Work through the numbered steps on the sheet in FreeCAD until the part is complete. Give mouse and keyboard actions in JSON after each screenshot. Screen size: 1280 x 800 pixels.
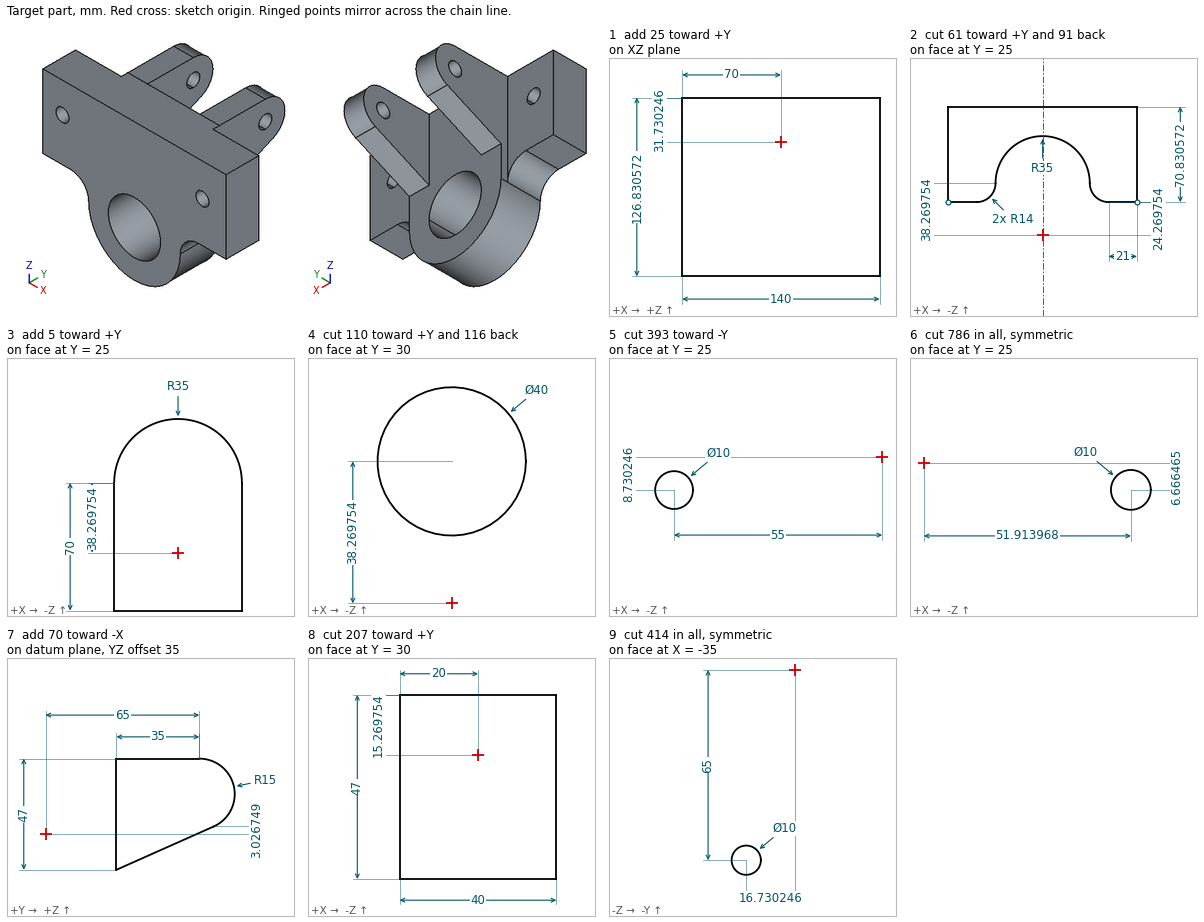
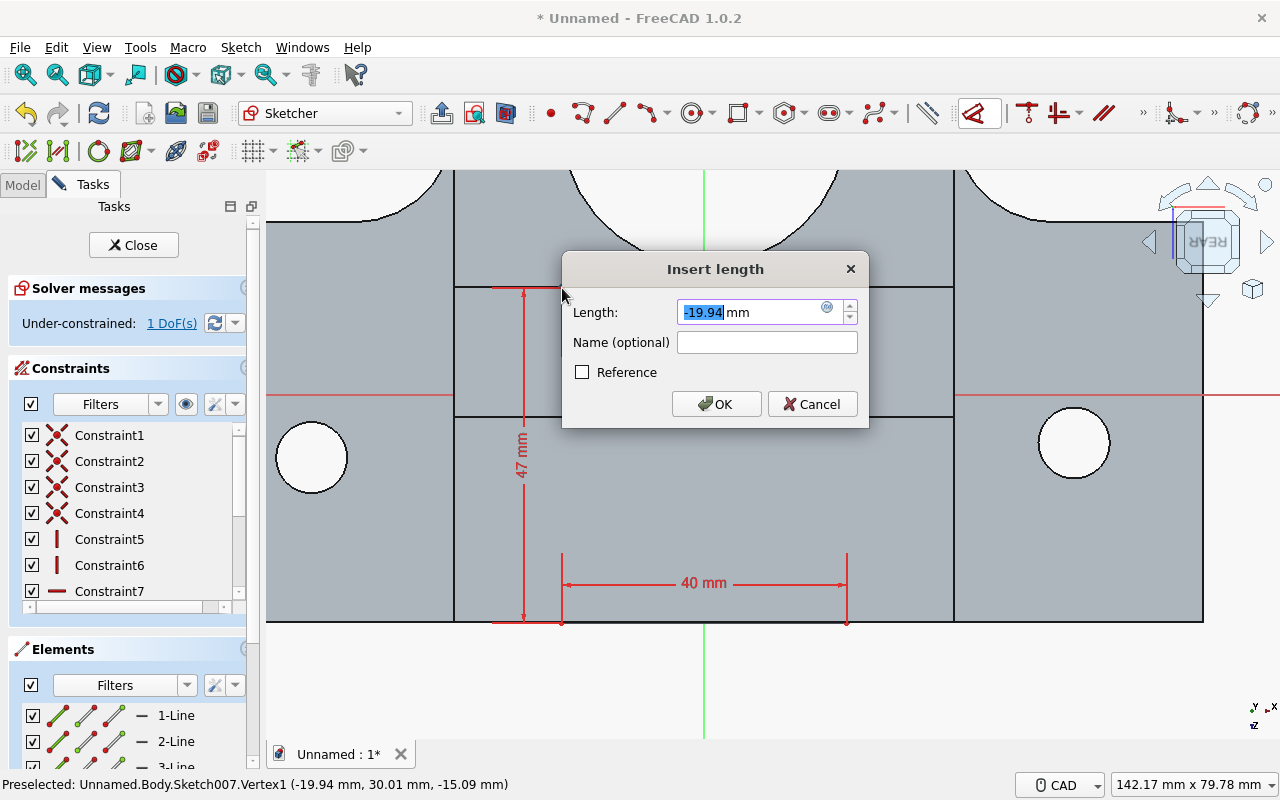
{"action": "type", "text": "-20"}
{"action": "key", "text": "Return"}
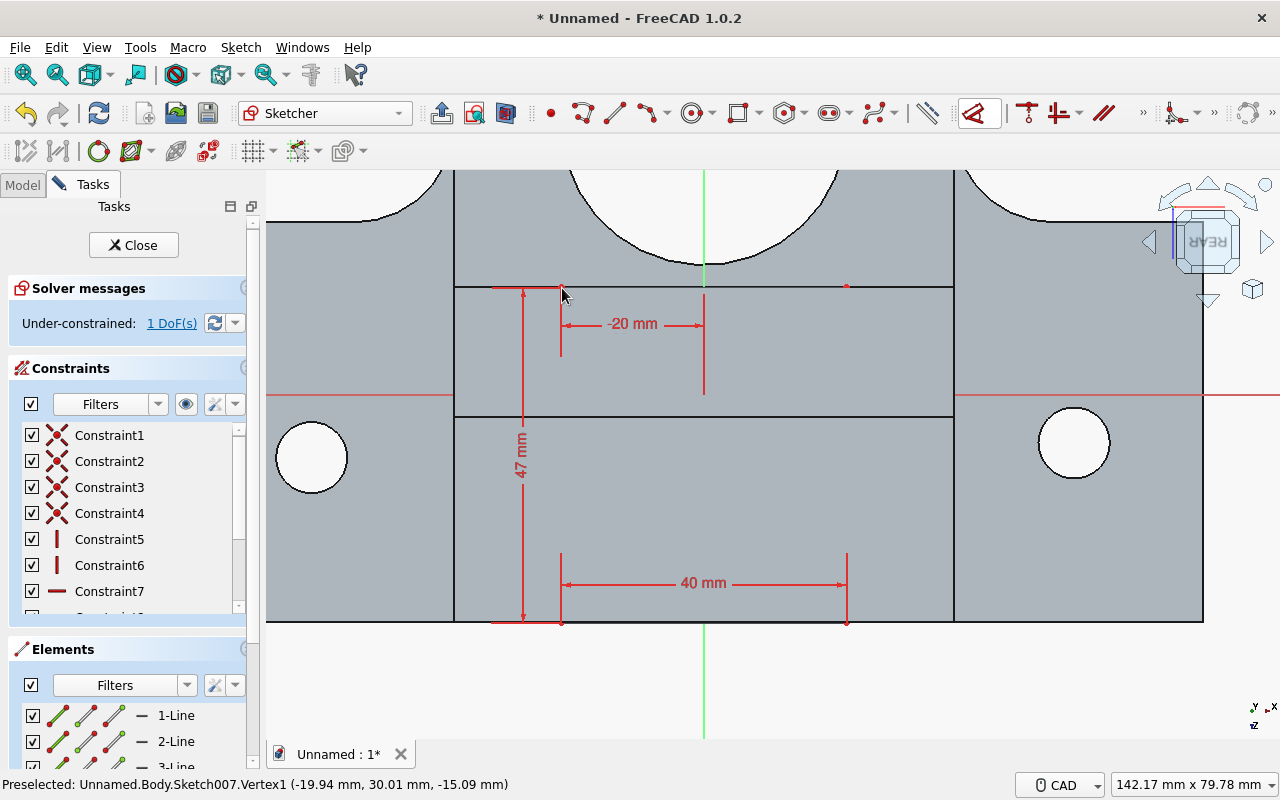
{"action": "left_click", "coordinate": [561, 288]}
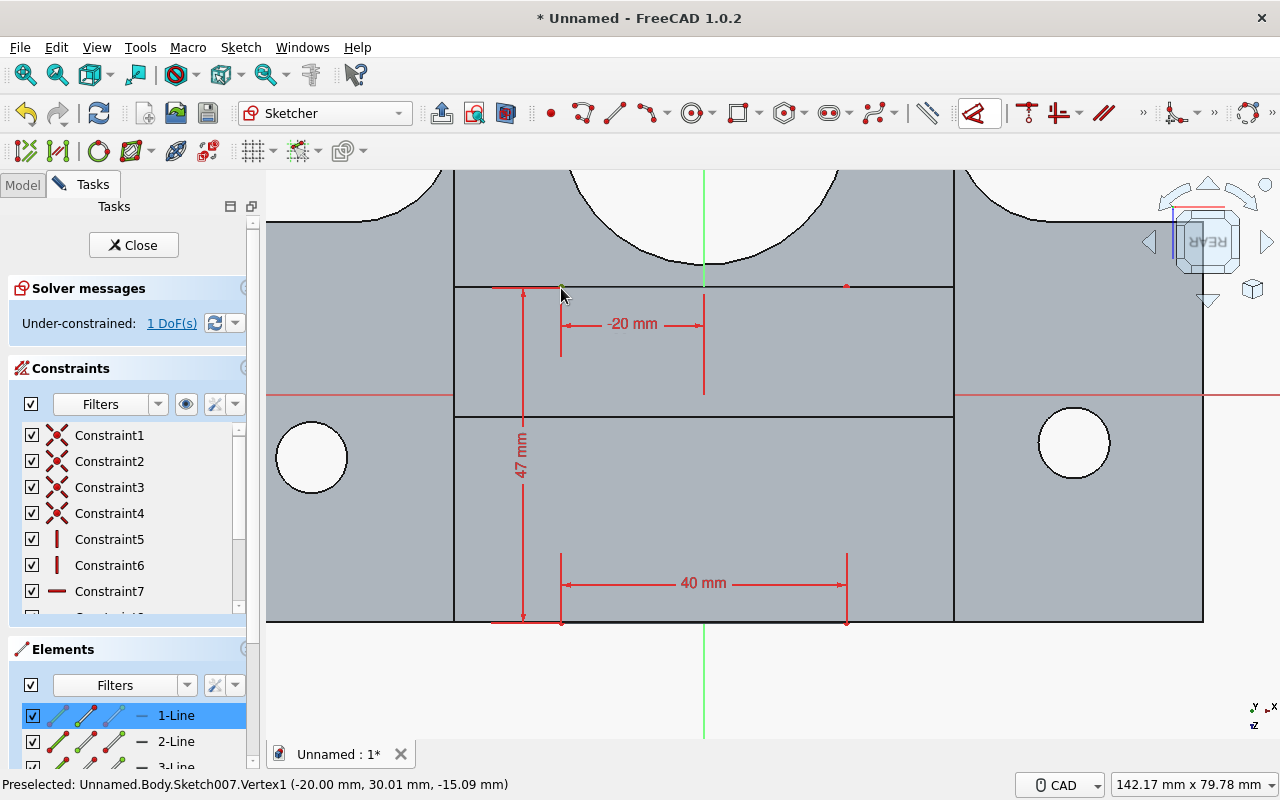
{"action": "key", "text": "i"}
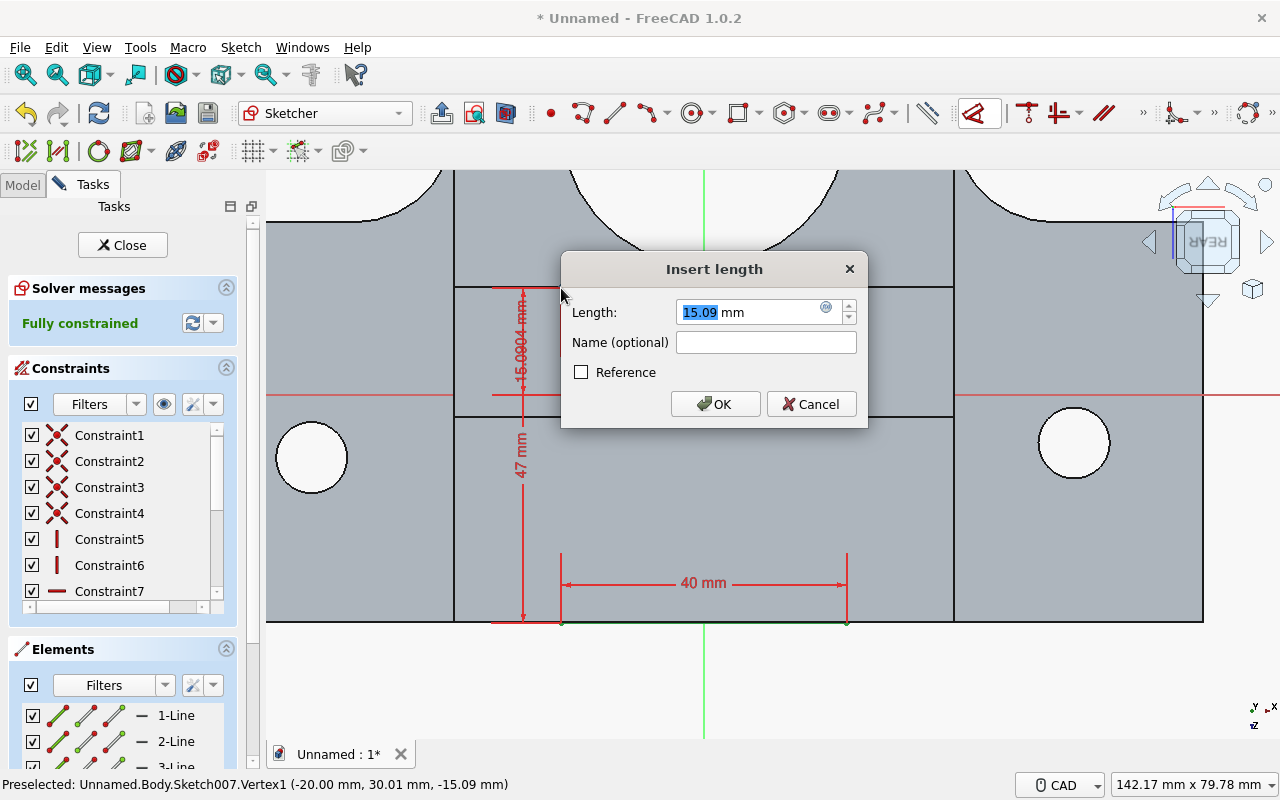
{"action": "type", "text": "15.269754"}
{"action": "key", "text": "Return"}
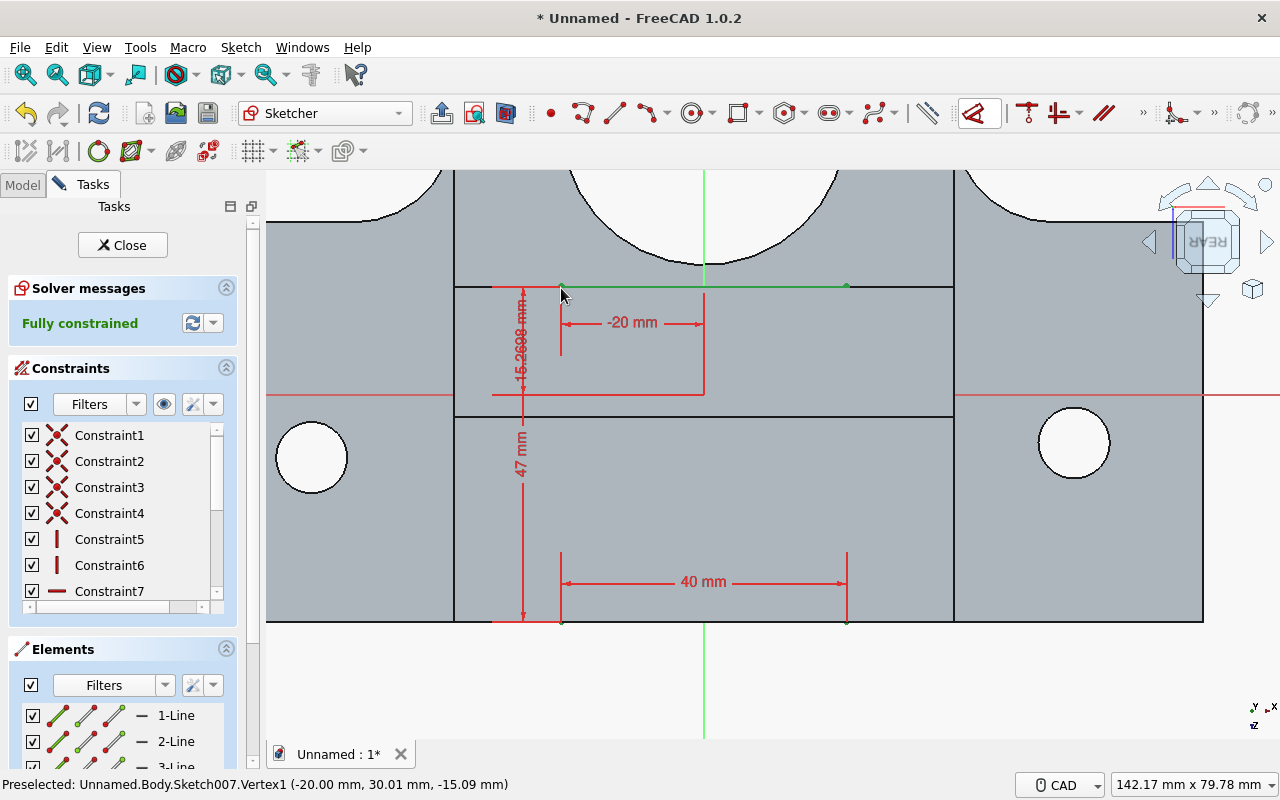
{"action": "left_click", "coordinate": [123, 245]}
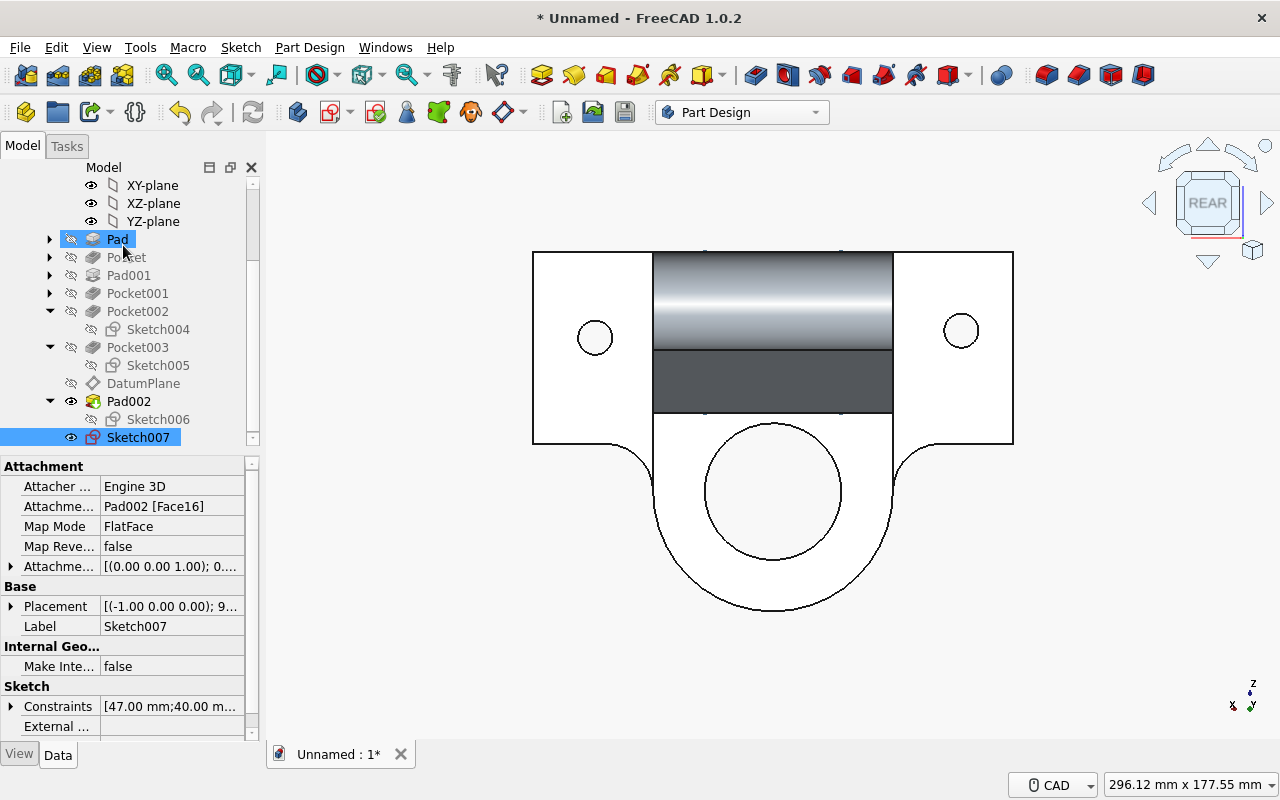
{"action": "left_click", "coordinate": [756, 76]}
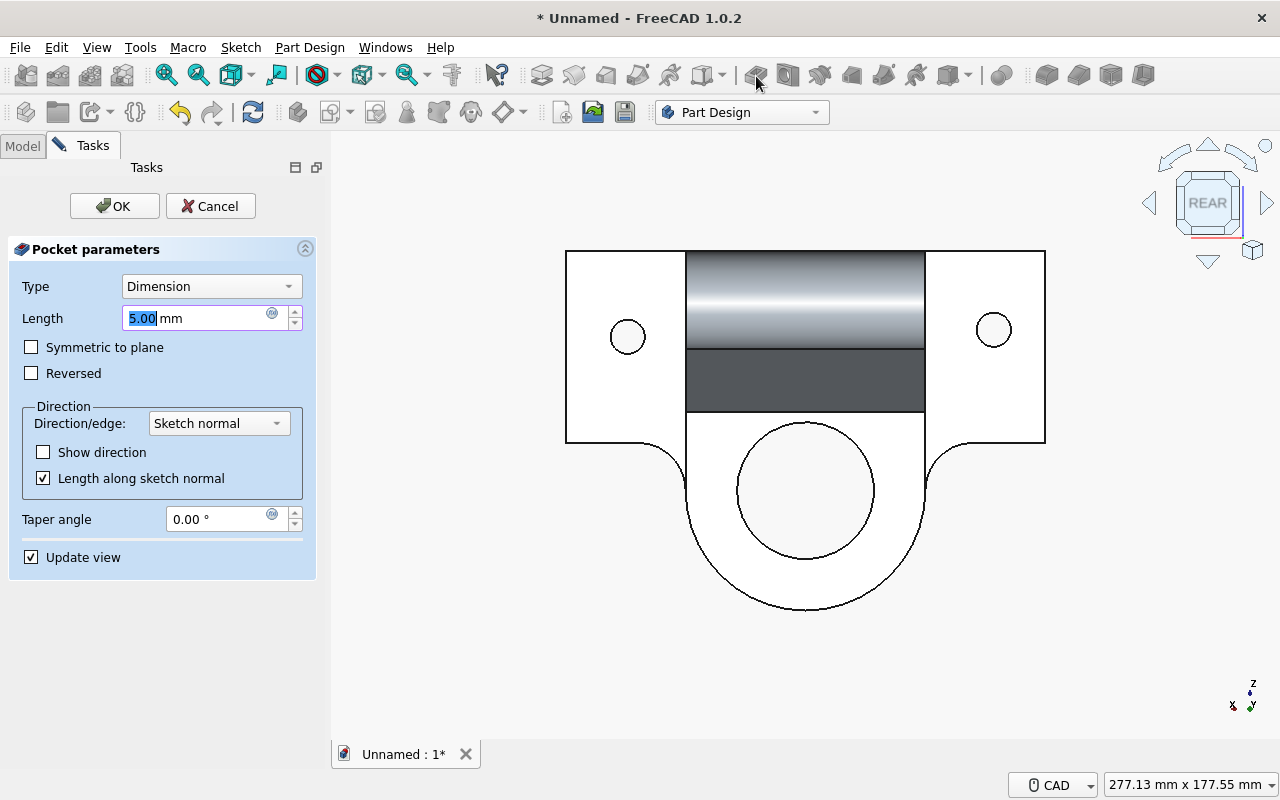
{"action": "type", "text": "207"}
{"action": "key", "text": "Tab"}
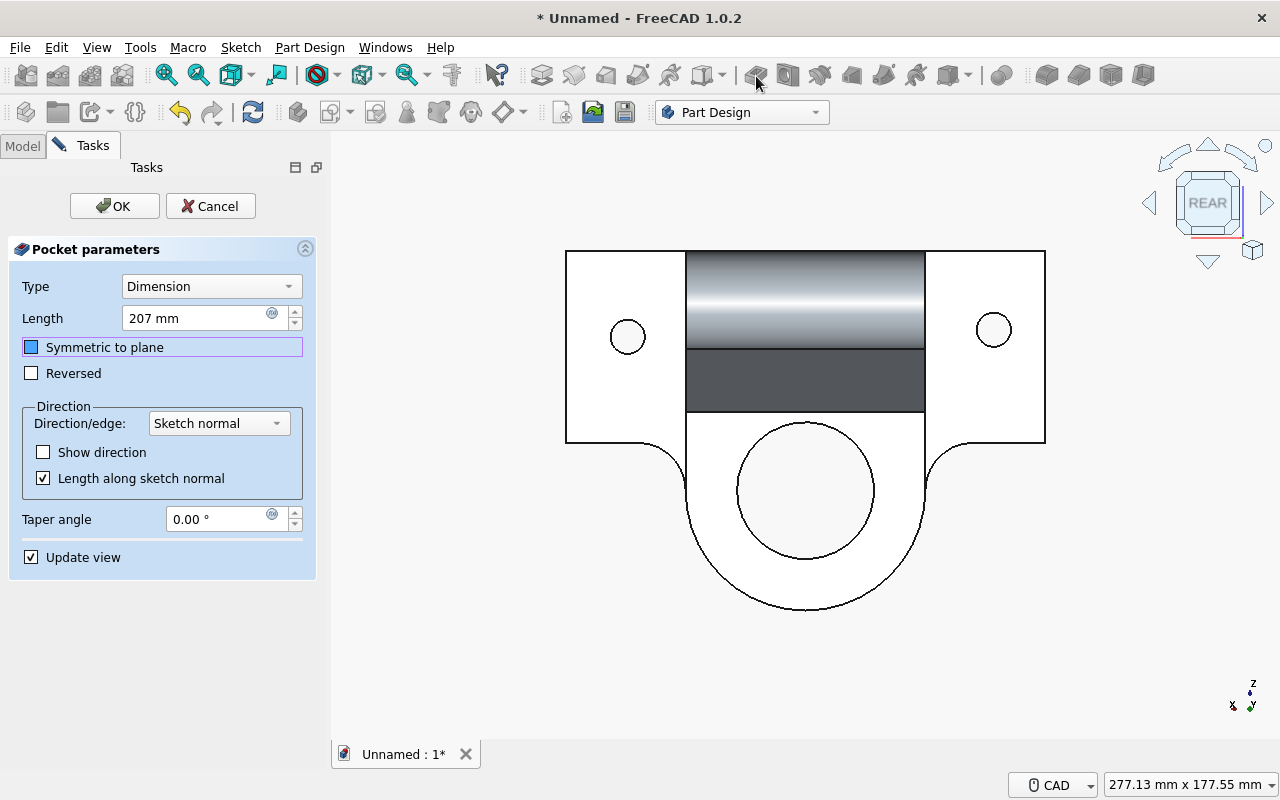
{"action": "left_click", "coordinate": [30, 373]}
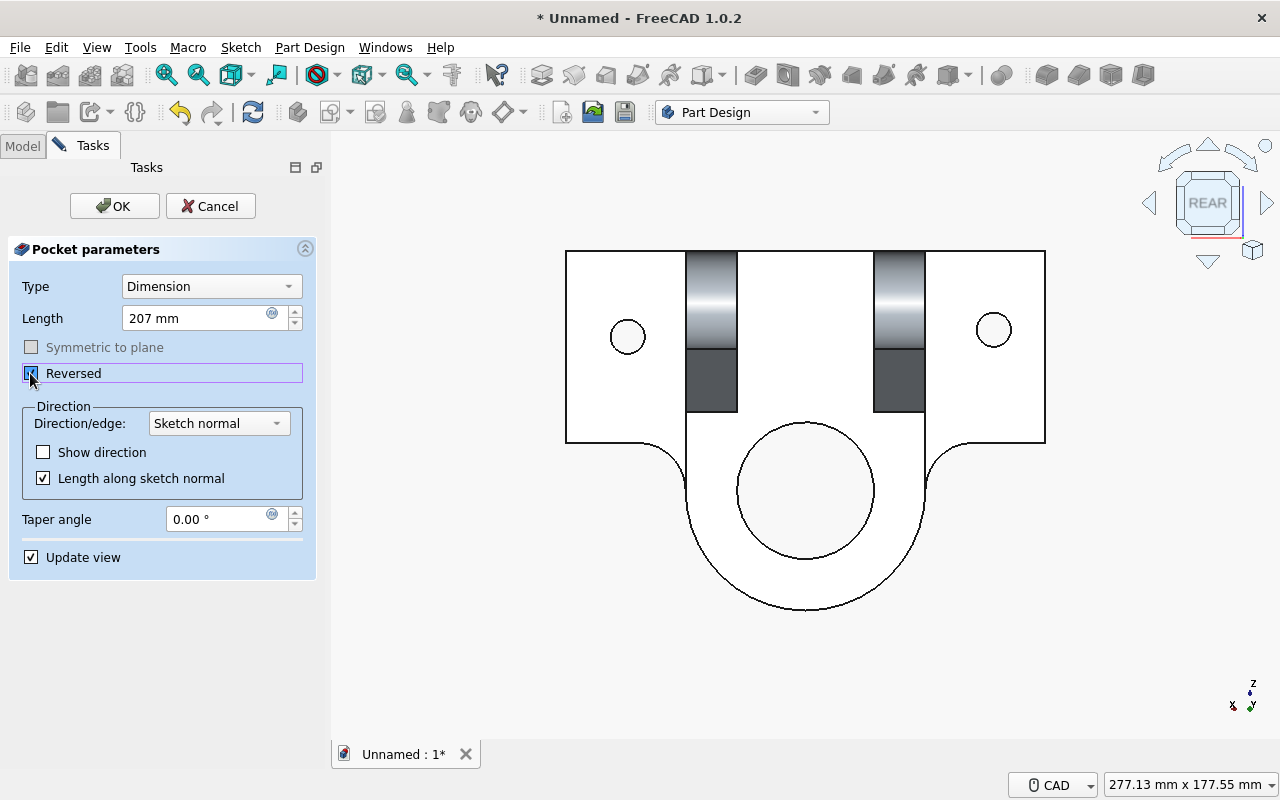
{"action": "left_click", "coordinate": [115, 206]}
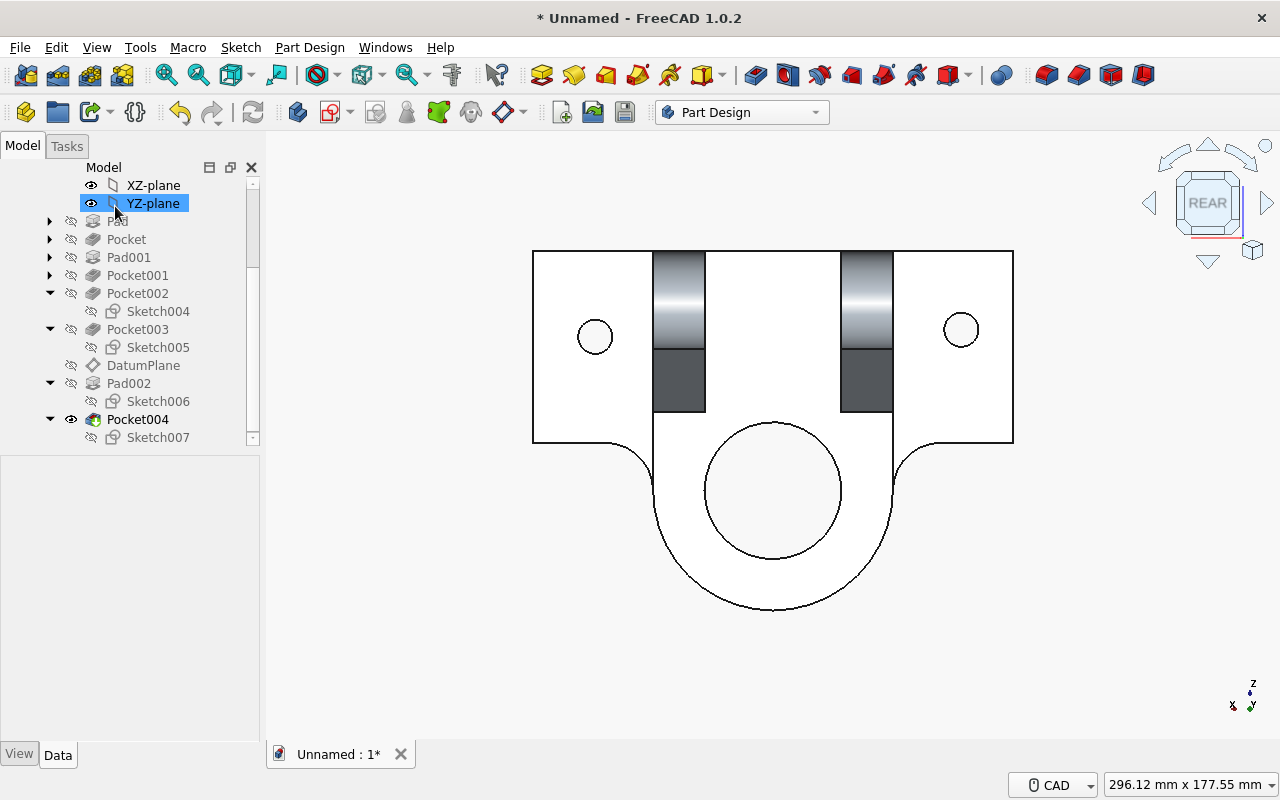
{"action": "key", "text": "6"}